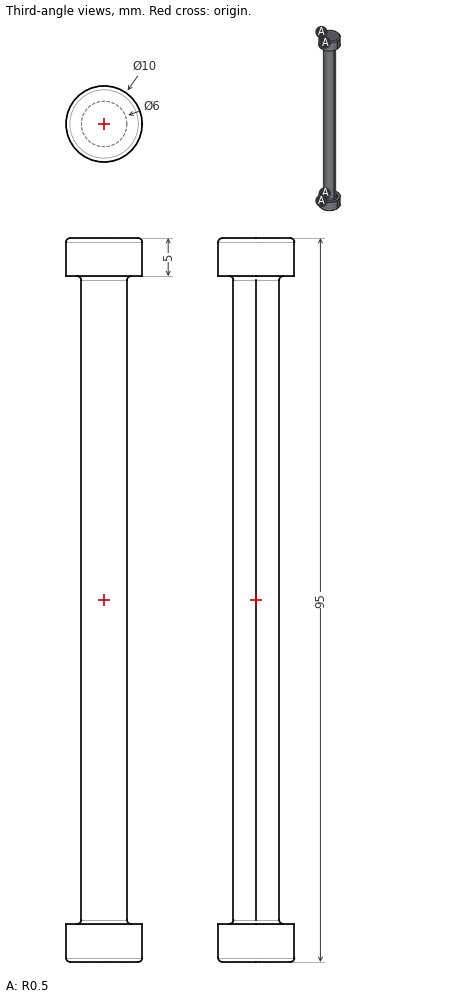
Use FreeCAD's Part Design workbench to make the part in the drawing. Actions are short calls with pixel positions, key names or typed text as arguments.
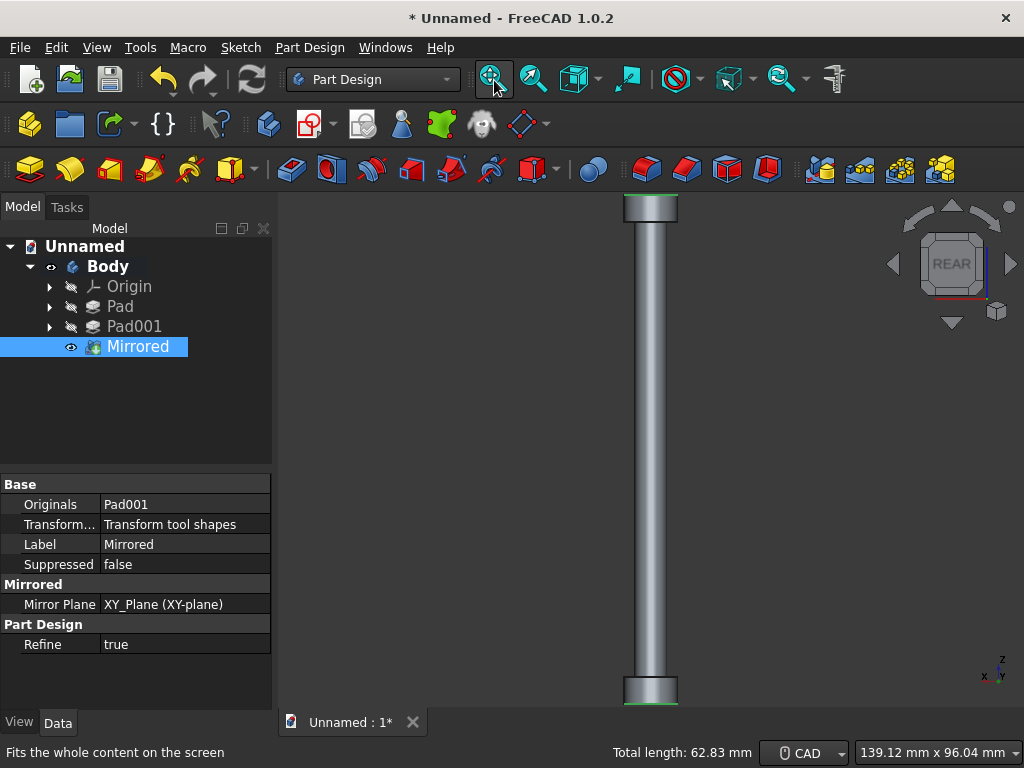
key(6)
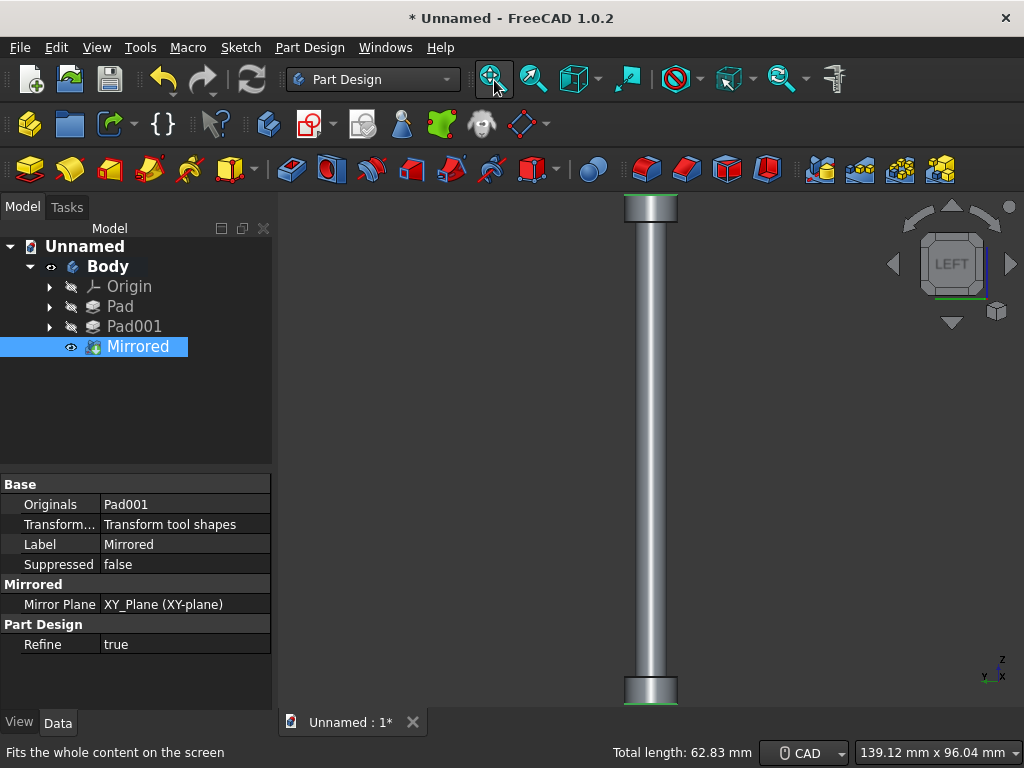
key(v)
key(3)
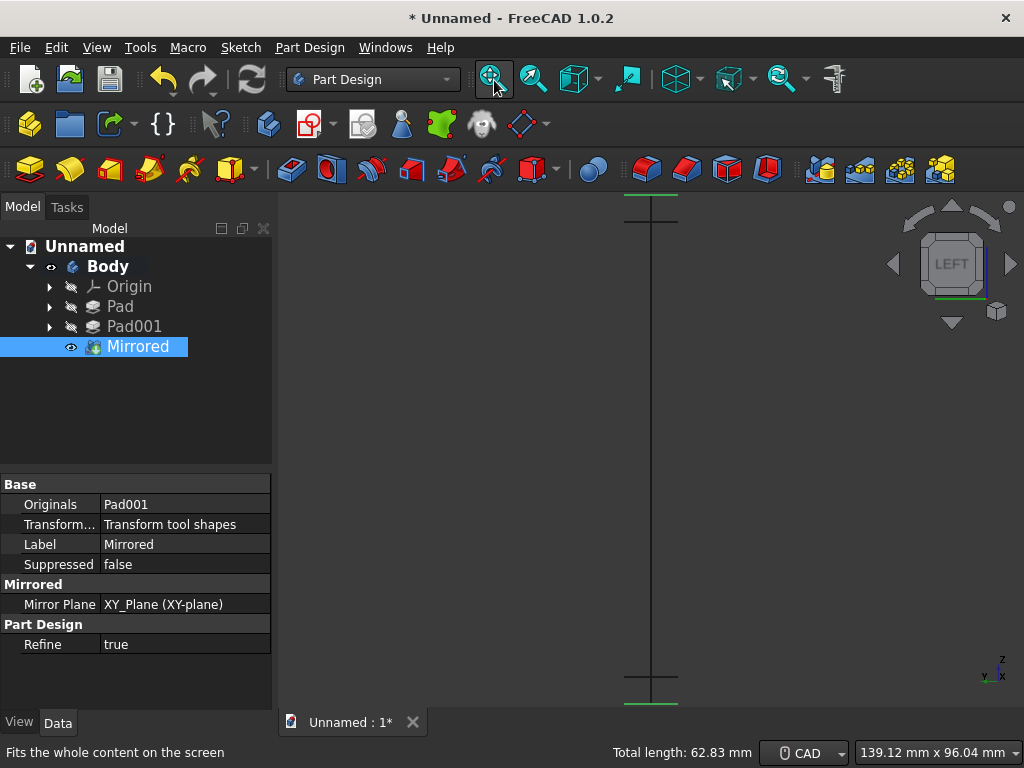
key(0)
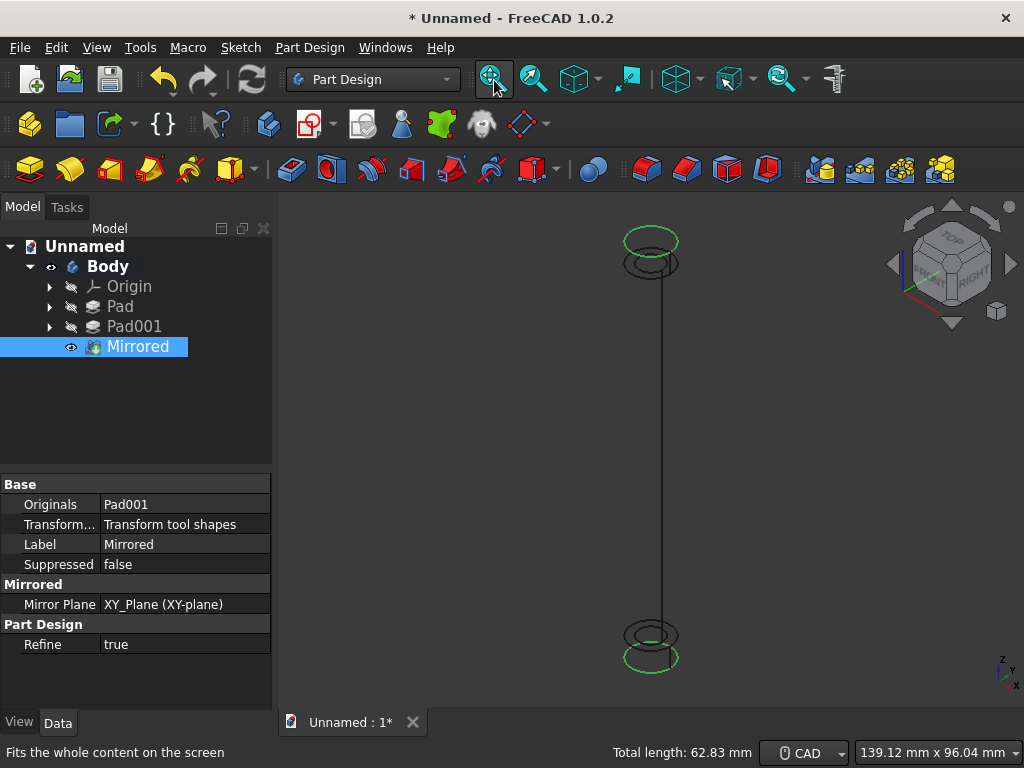
click(640, 628, ctrl)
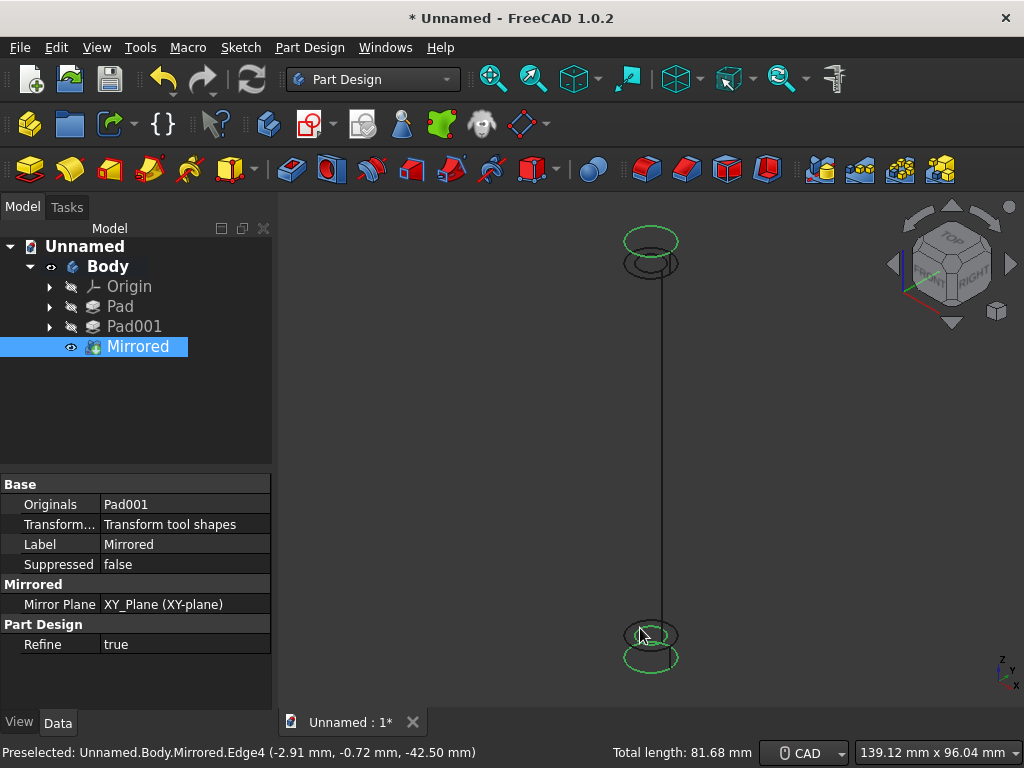
click(635, 261, ctrl)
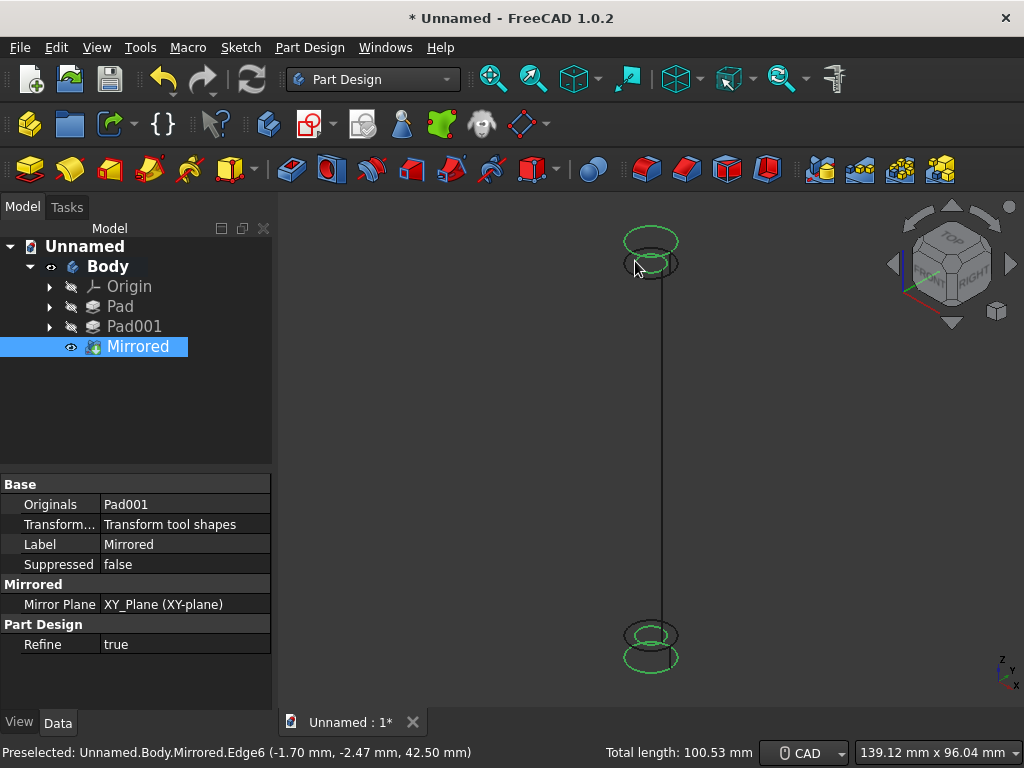
key(v)
key(1)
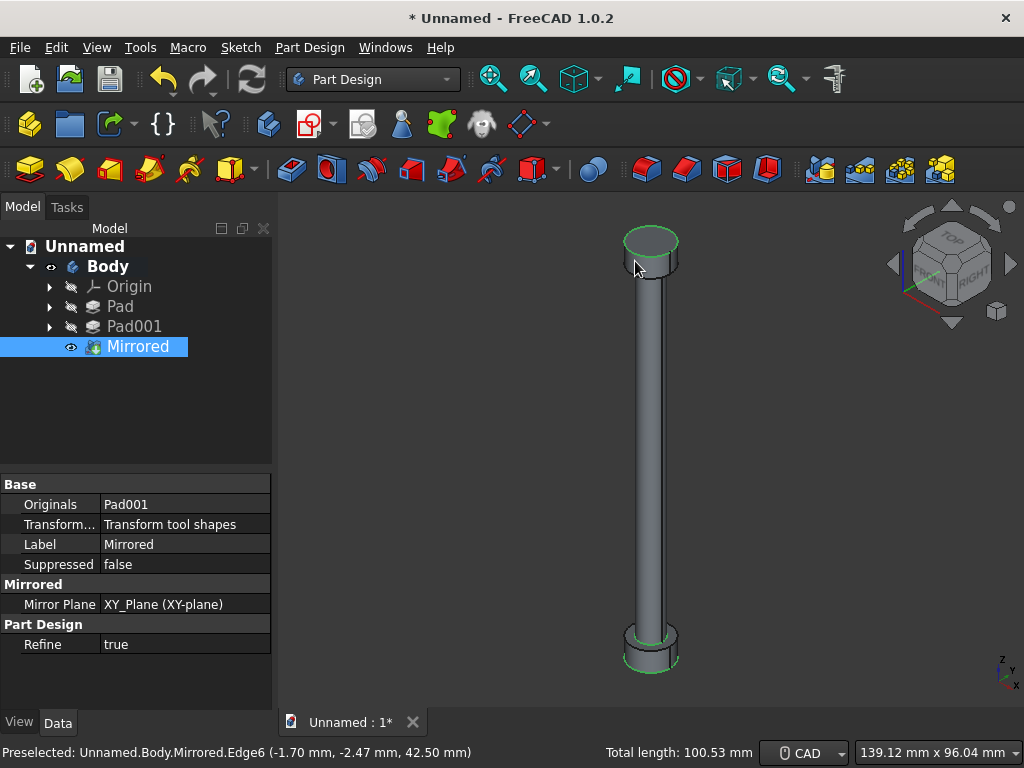
click(648, 170)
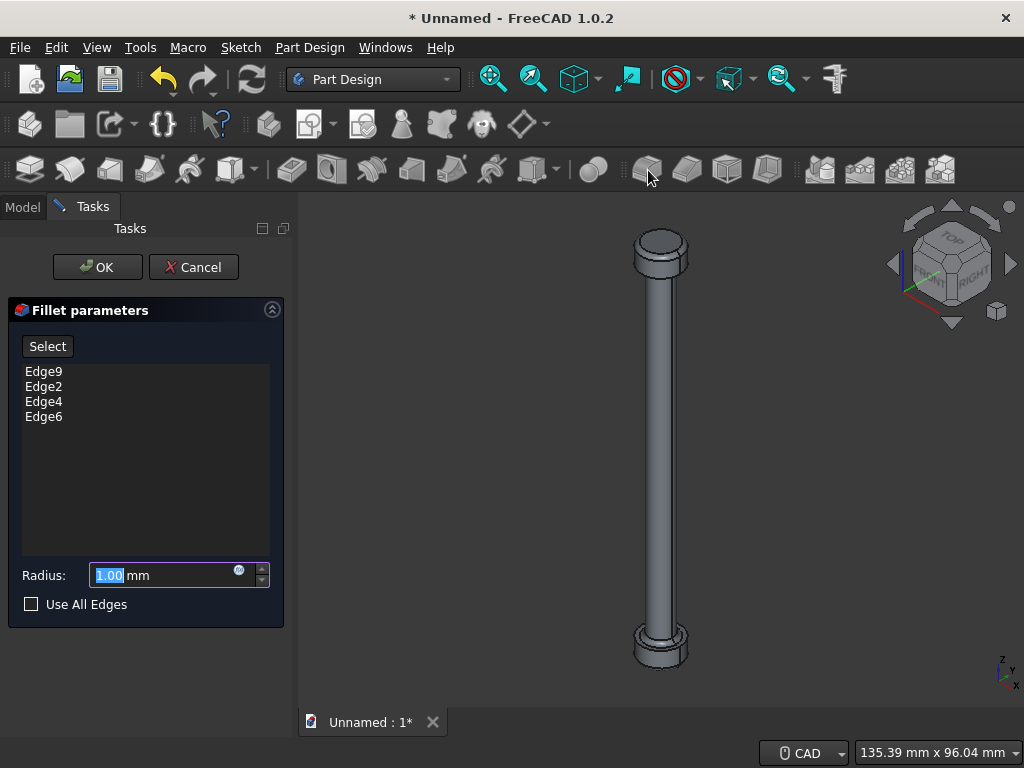
text(0.5)
key(Tab)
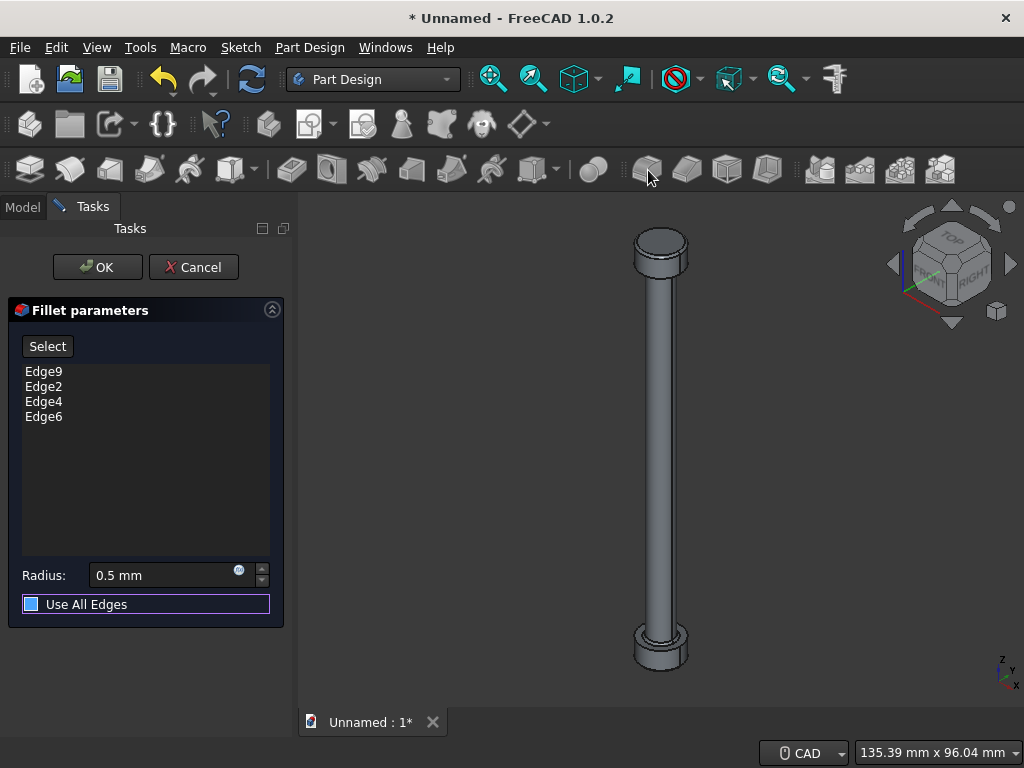
click(98, 267)